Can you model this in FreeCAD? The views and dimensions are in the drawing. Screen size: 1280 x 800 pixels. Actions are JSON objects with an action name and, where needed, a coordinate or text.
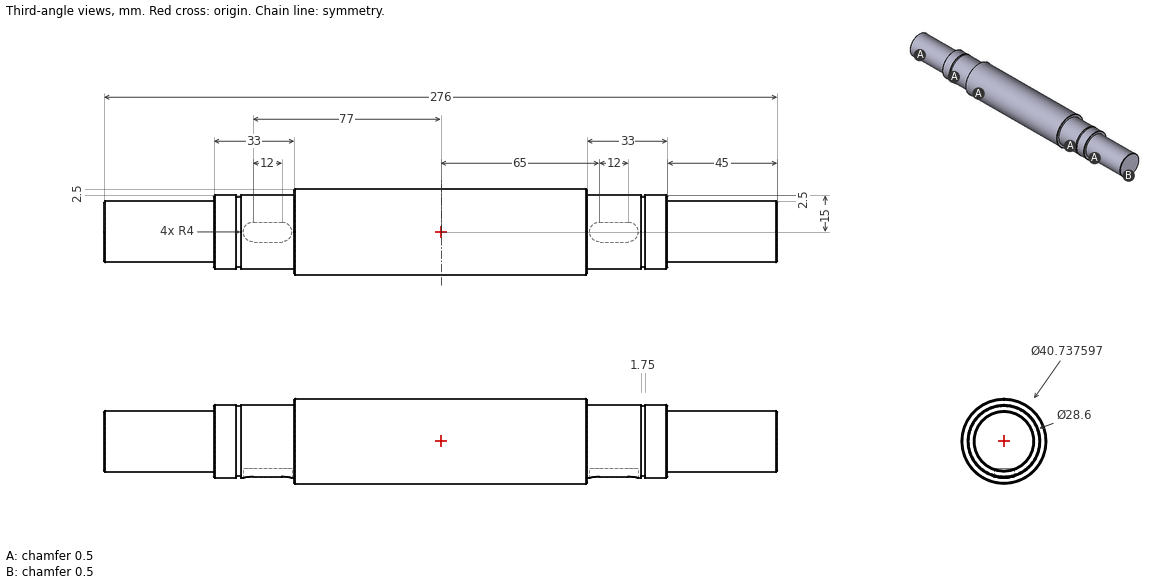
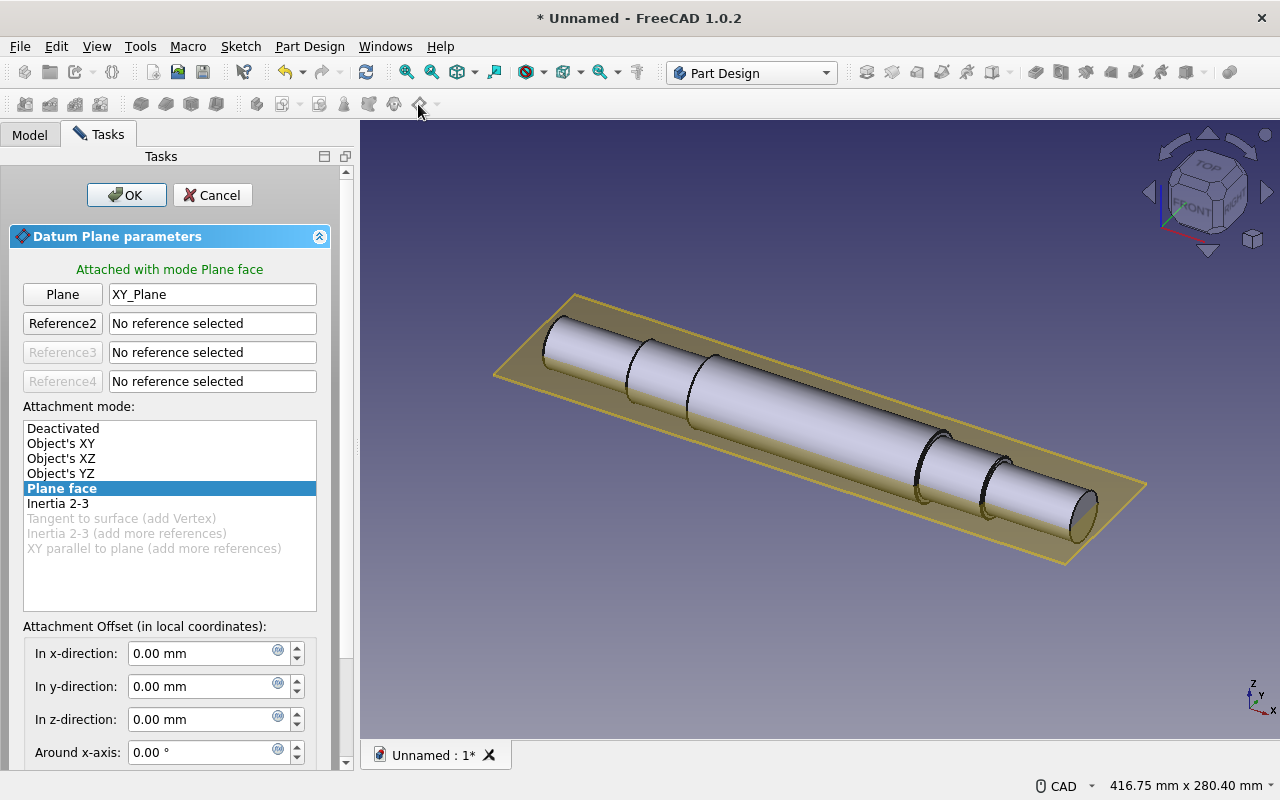
{"action": "triple_click", "coordinate": [210, 720]}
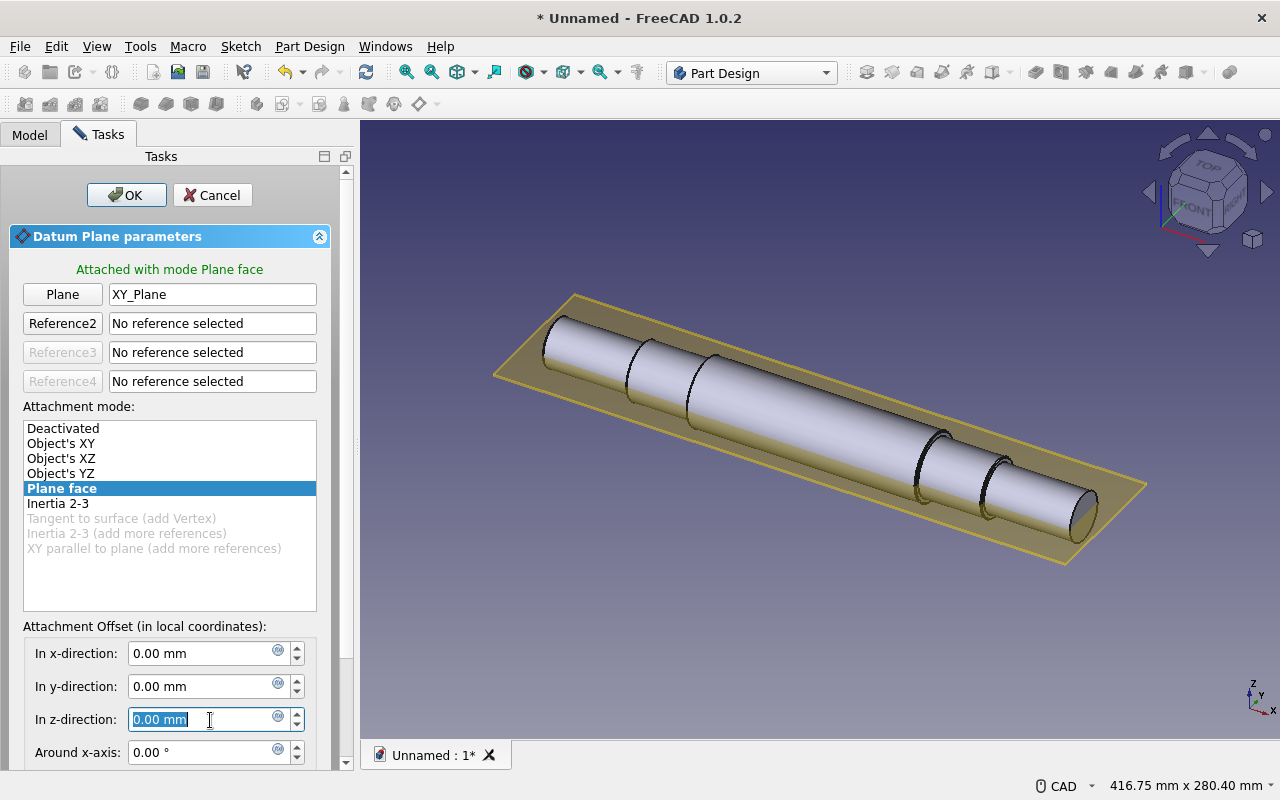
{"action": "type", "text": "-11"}
{"action": "key", "text": "Tab"}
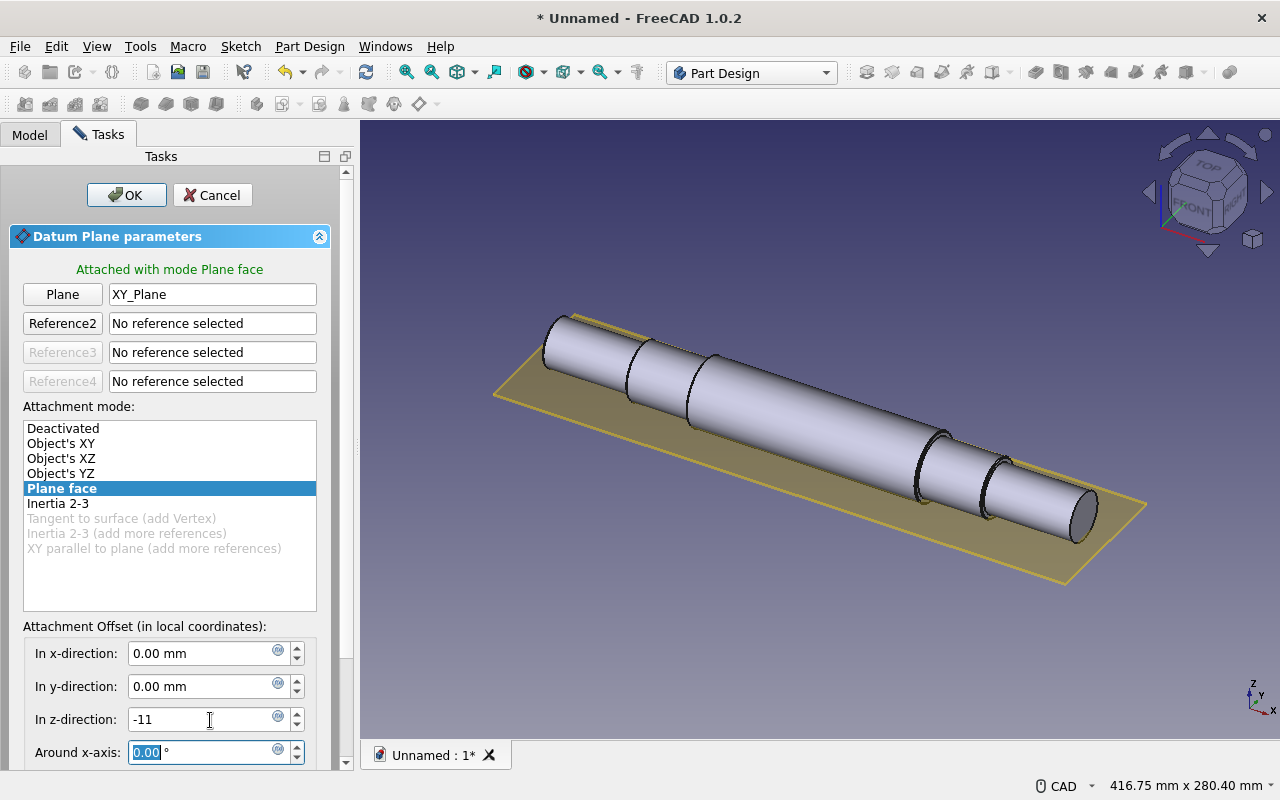
{"action": "left_click", "coordinate": [127, 195]}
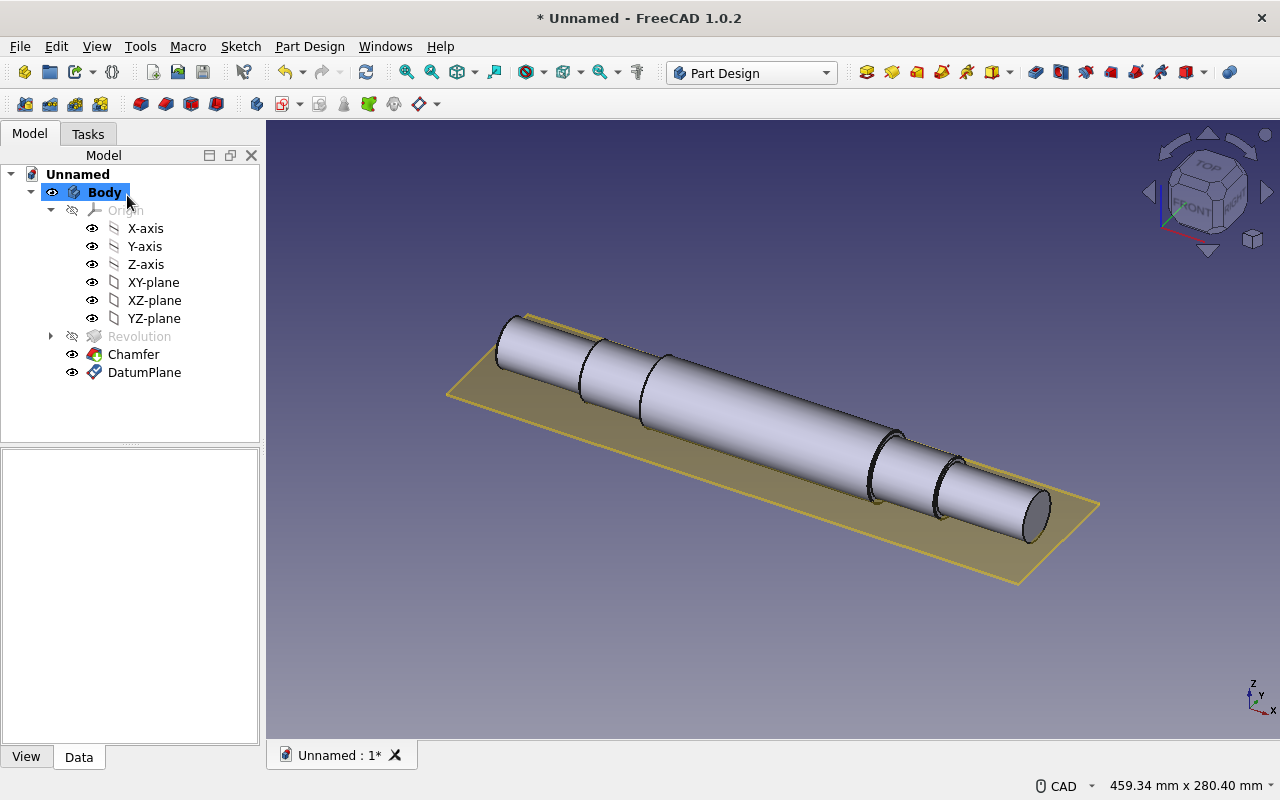
{"action": "left_click", "coordinate": [117, 372]}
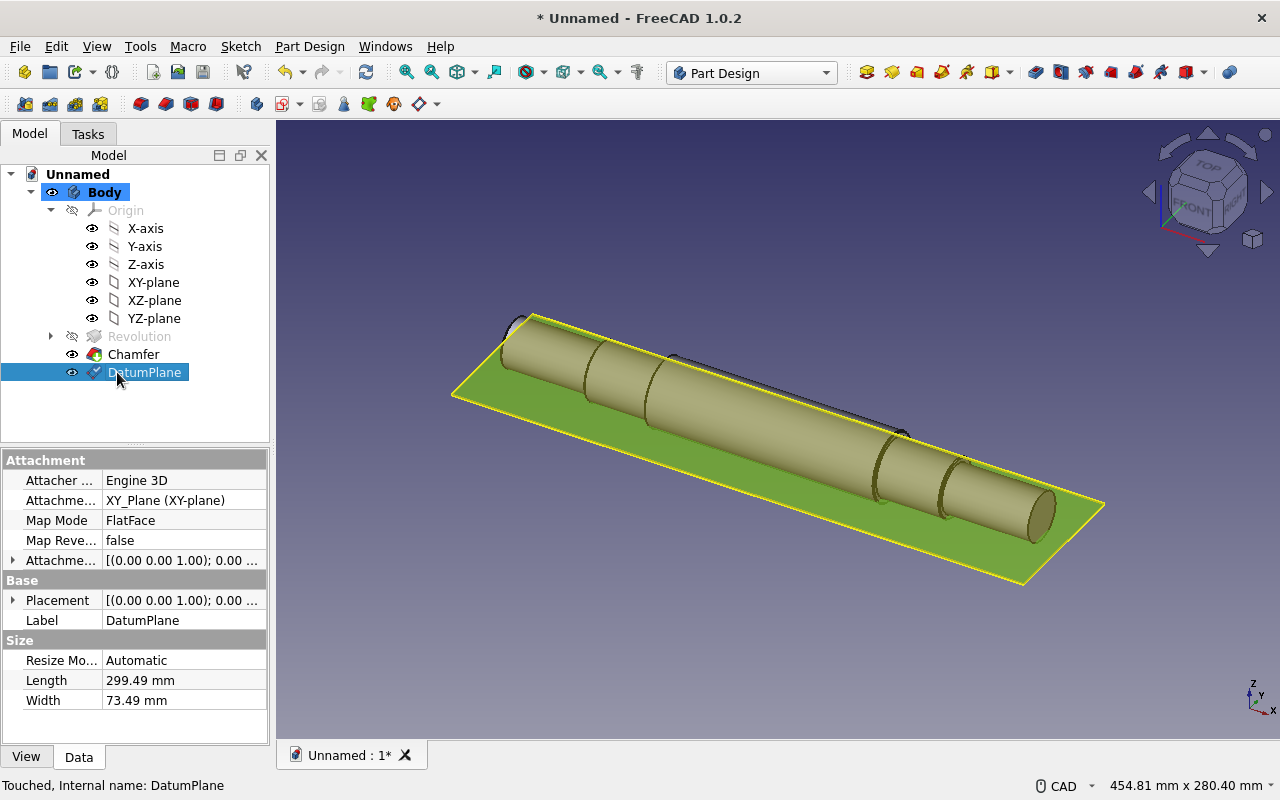
{"action": "left_click", "coordinate": [282, 104]}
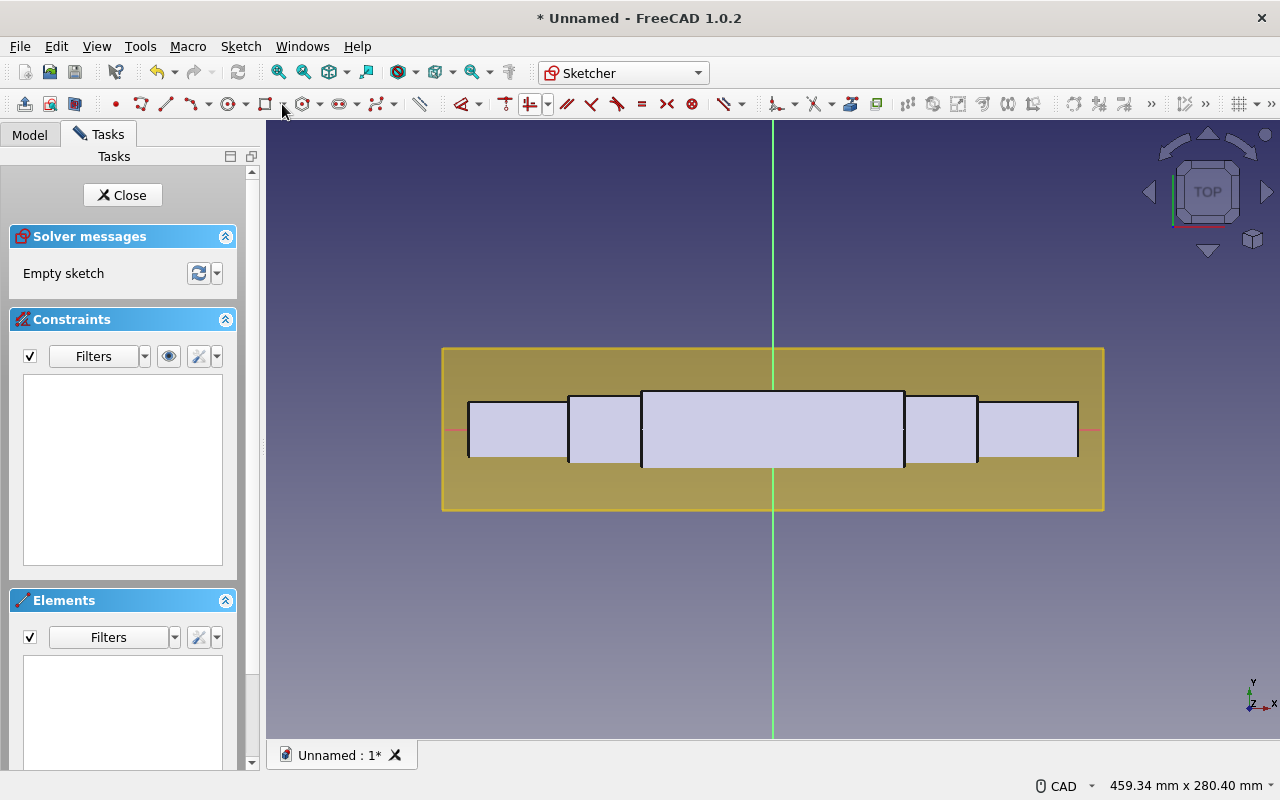
{"action": "left_click", "coordinate": [75, 104]}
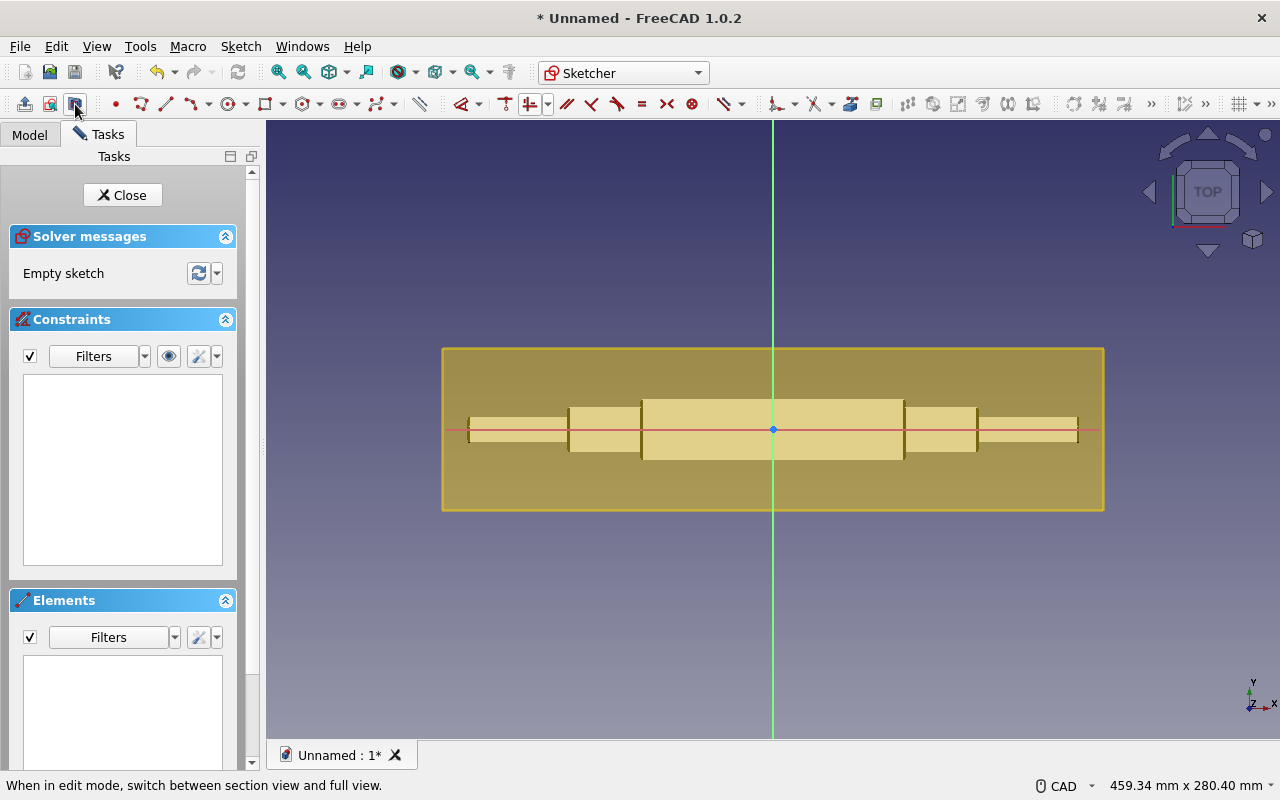
{"action": "scroll", "coordinate": [912, 429], "scroll_direction": "up", "scroll_amount": 2}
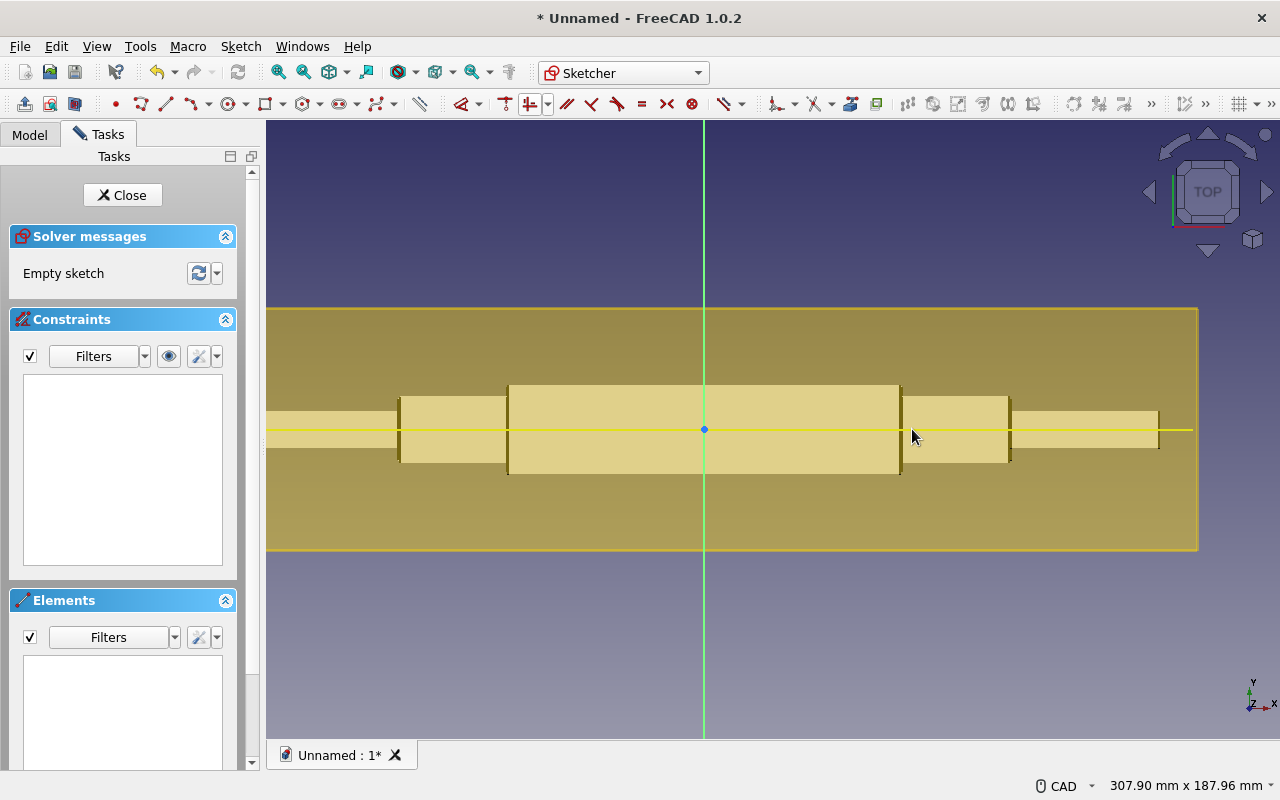
{"action": "left_click", "coordinate": [338, 104]}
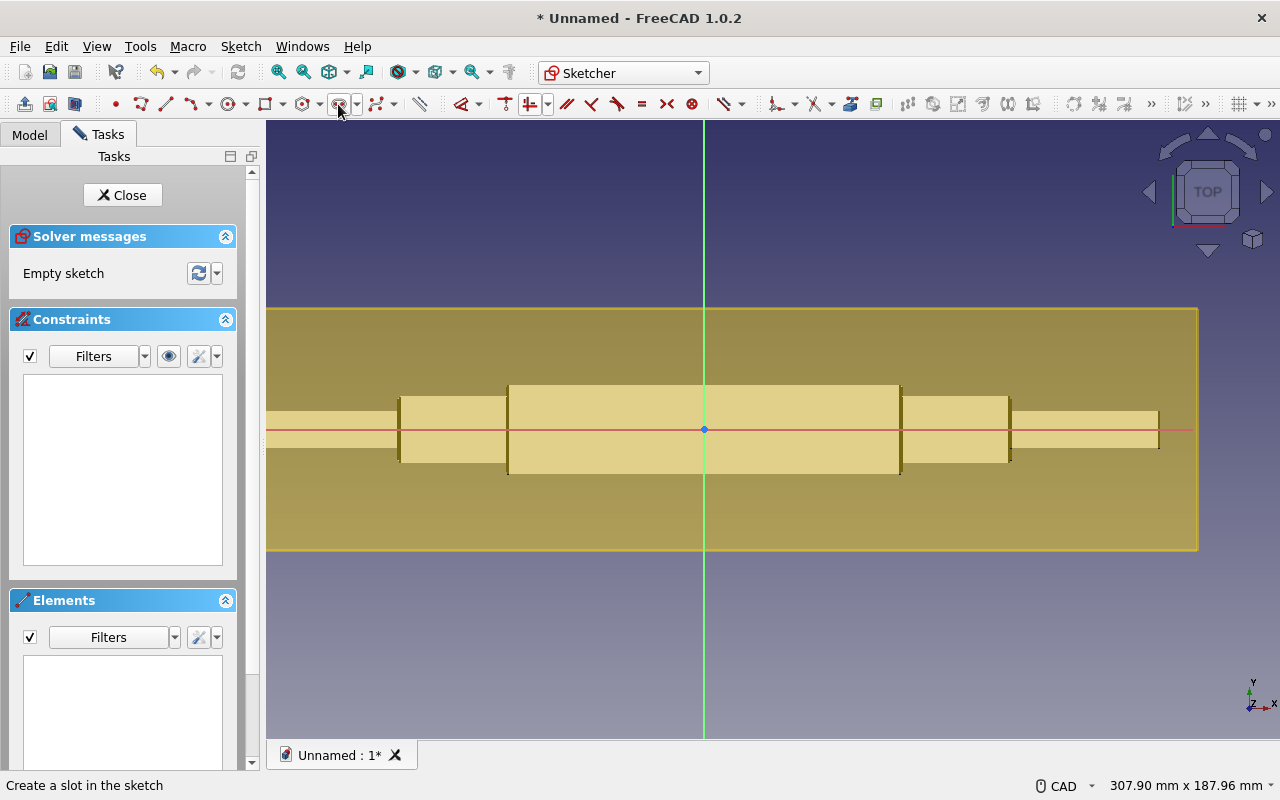
{"action": "scroll", "coordinate": [451, 430], "scroll_direction": "up", "scroll_amount": 3}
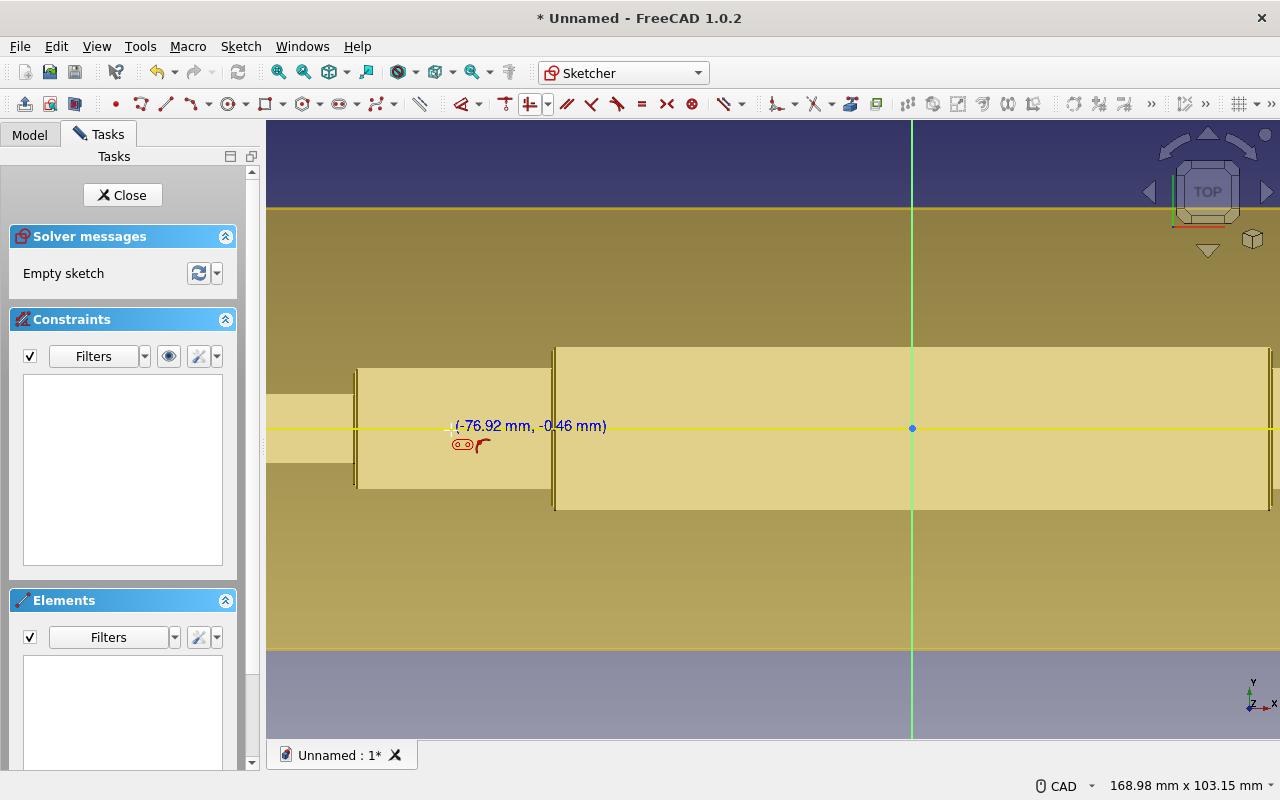
{"action": "left_click", "coordinate": [450, 429]}